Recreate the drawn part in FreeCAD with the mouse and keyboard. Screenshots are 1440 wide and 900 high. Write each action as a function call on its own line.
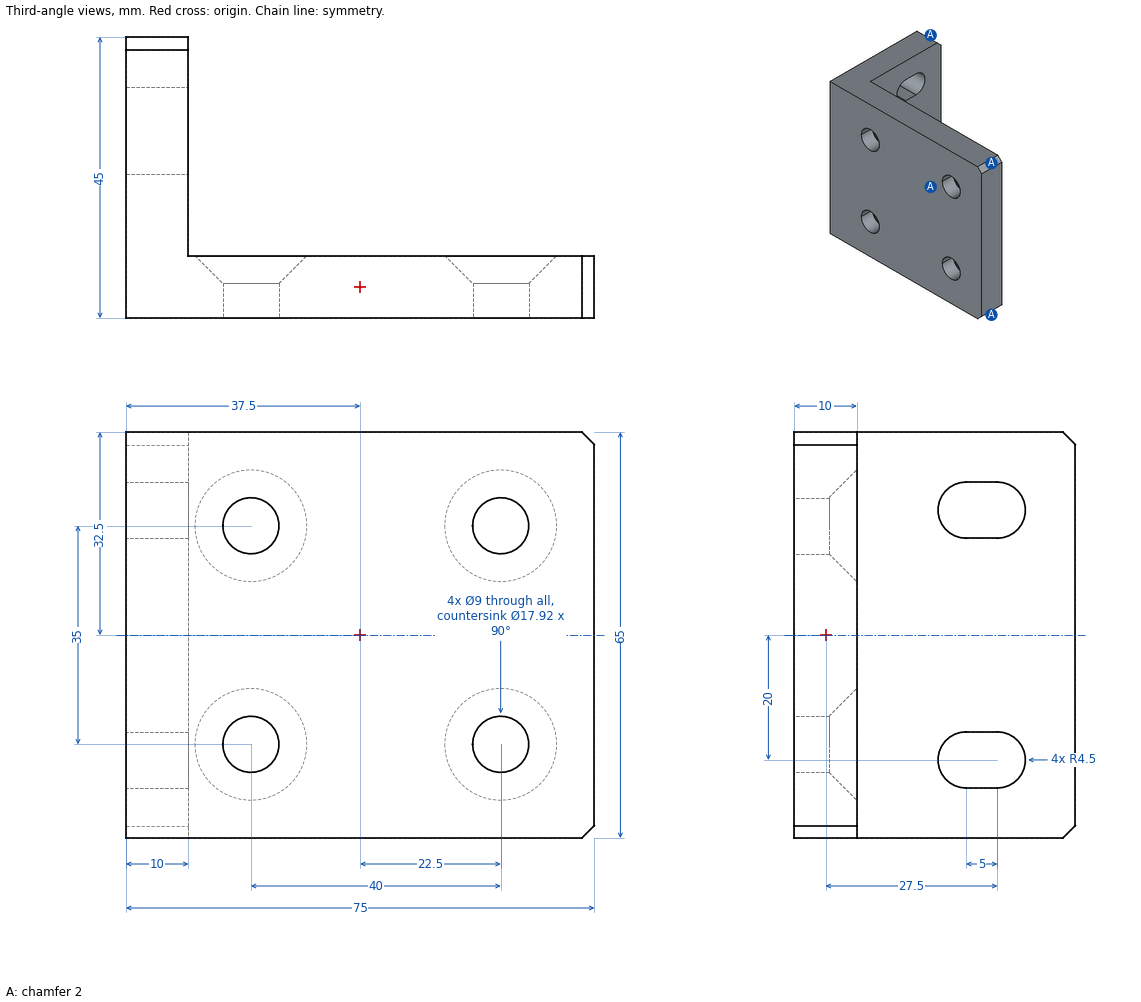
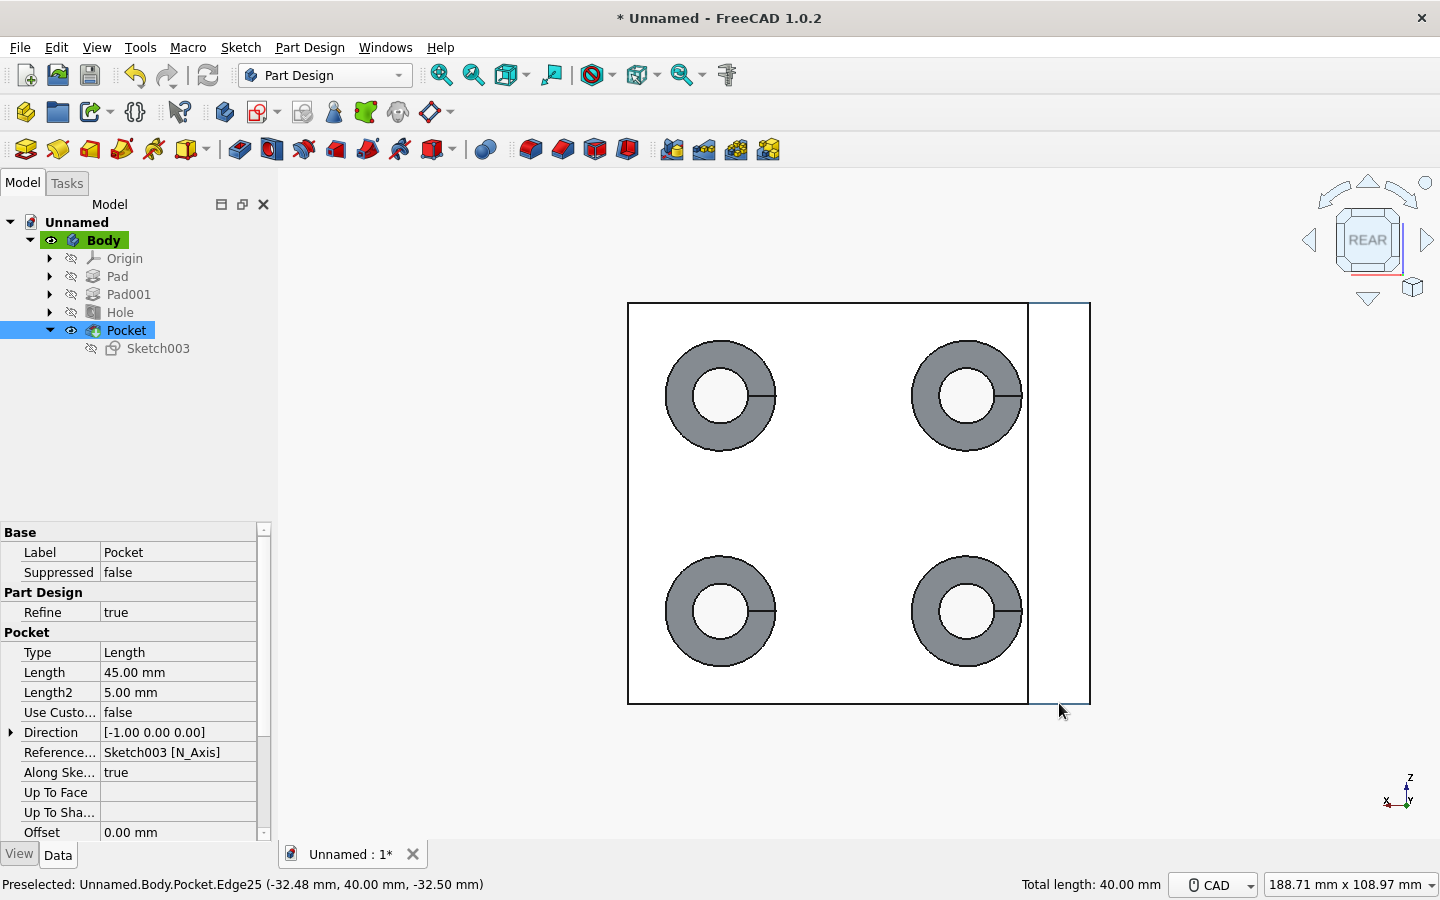
click(564, 150)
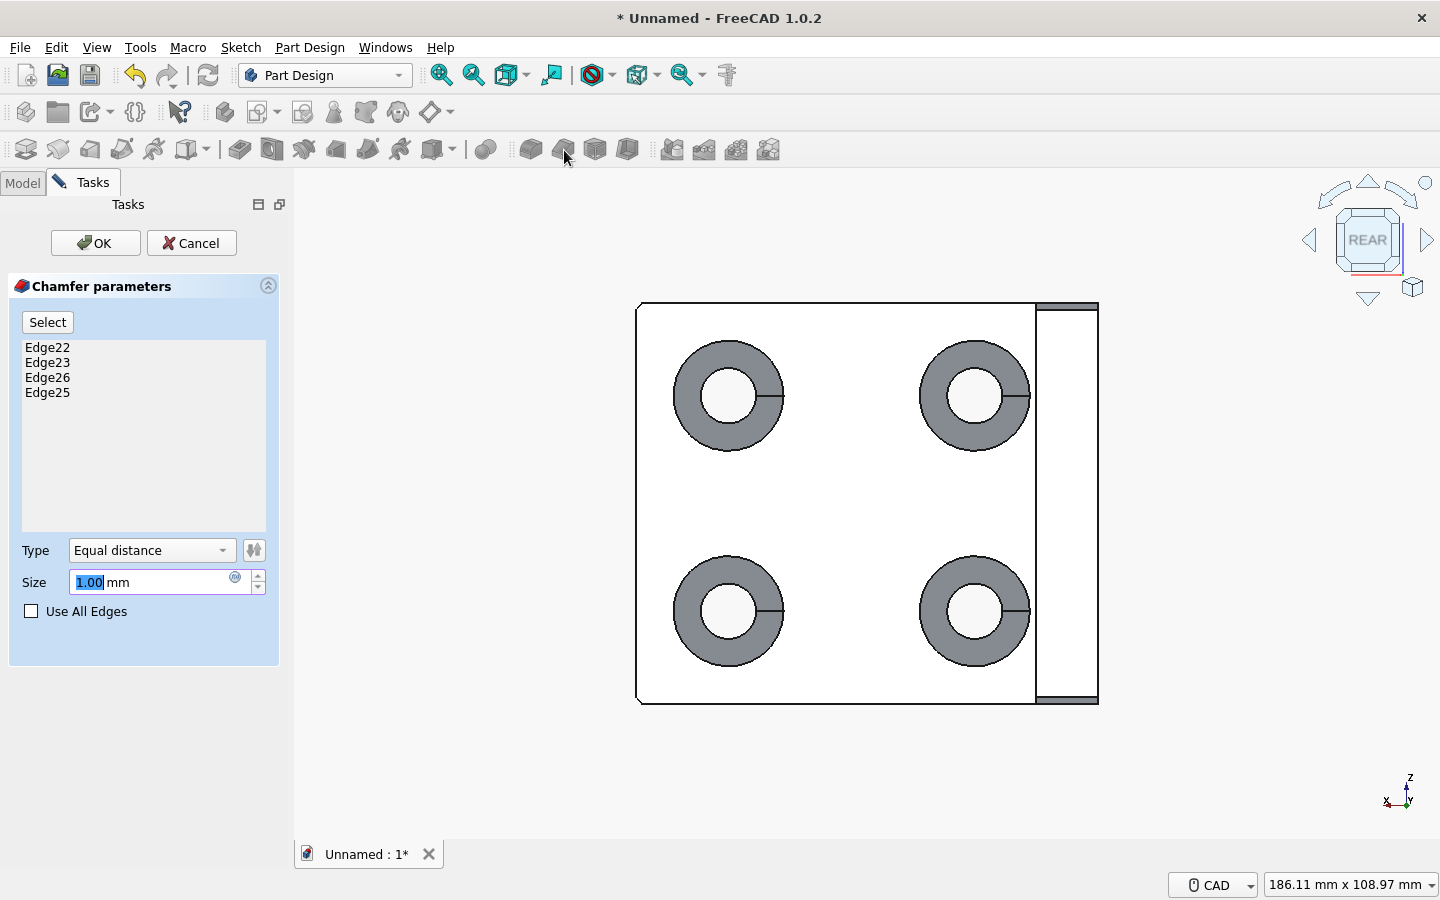
text(2)
key(Tab)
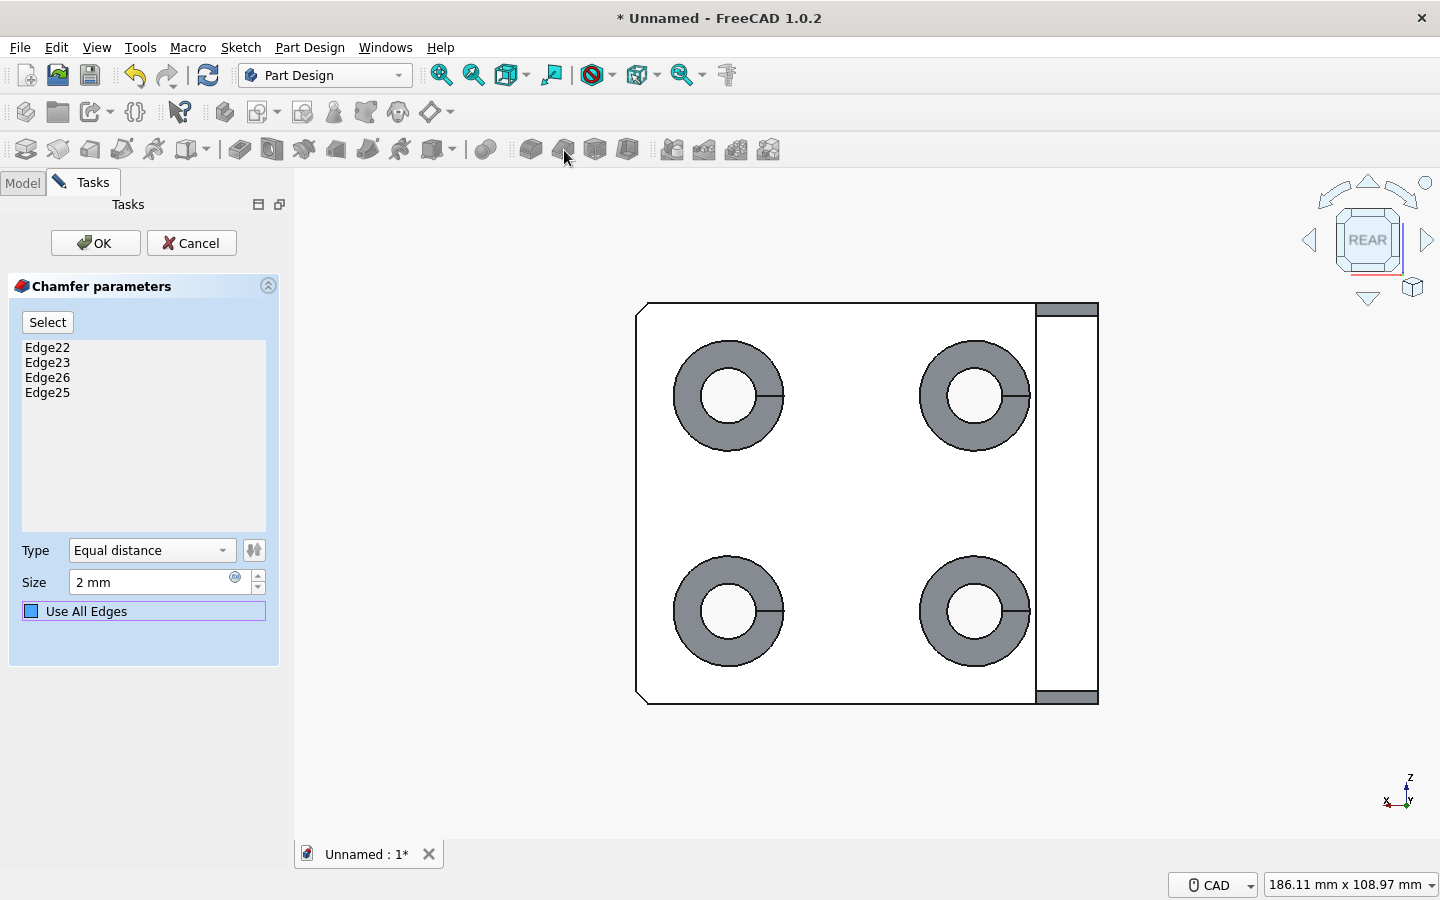
click(96, 243)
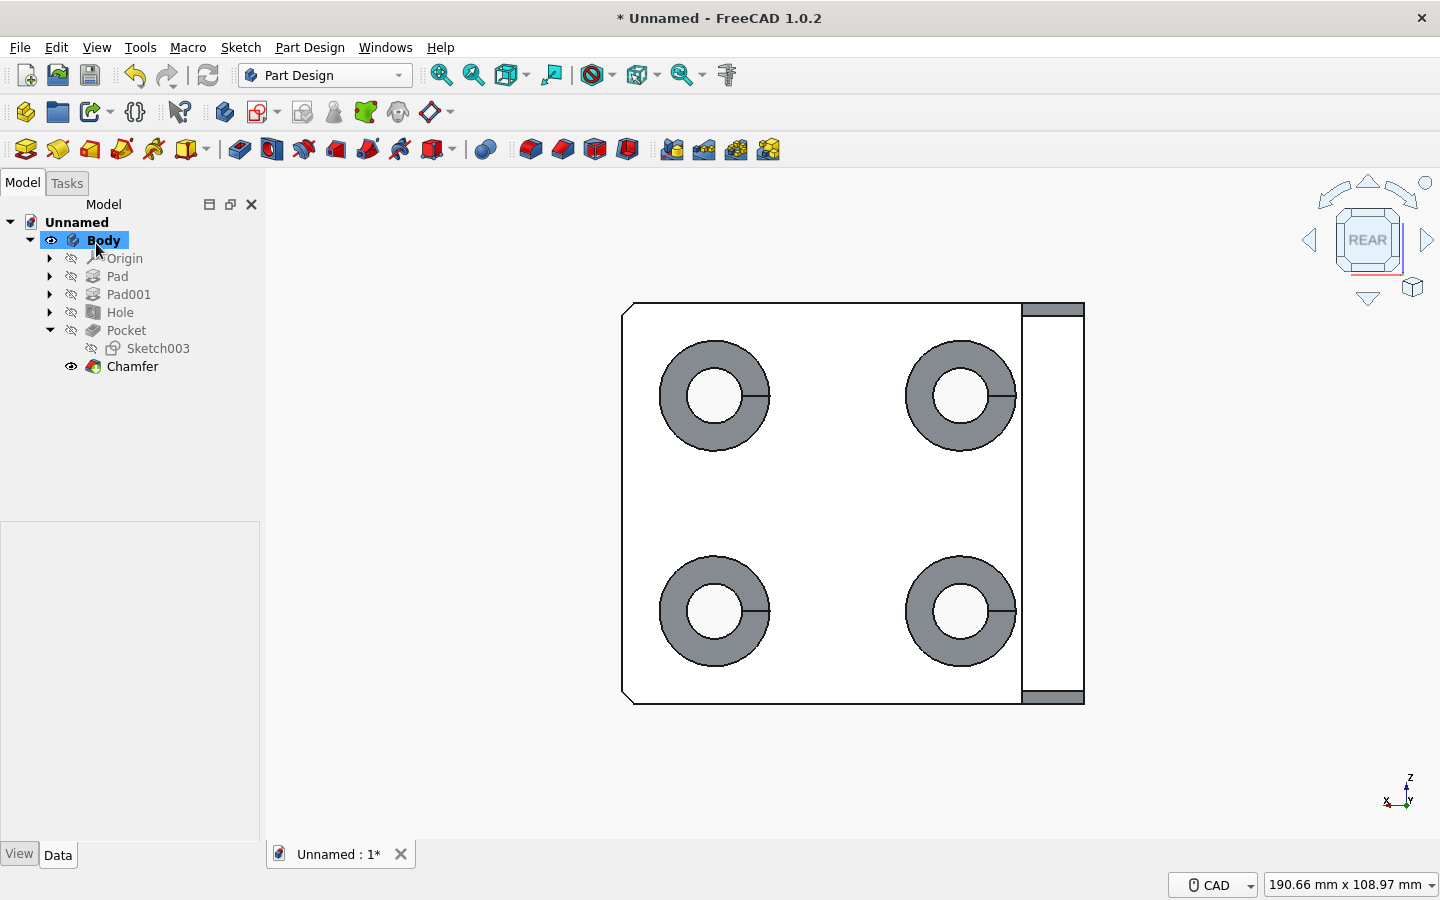
key(0)